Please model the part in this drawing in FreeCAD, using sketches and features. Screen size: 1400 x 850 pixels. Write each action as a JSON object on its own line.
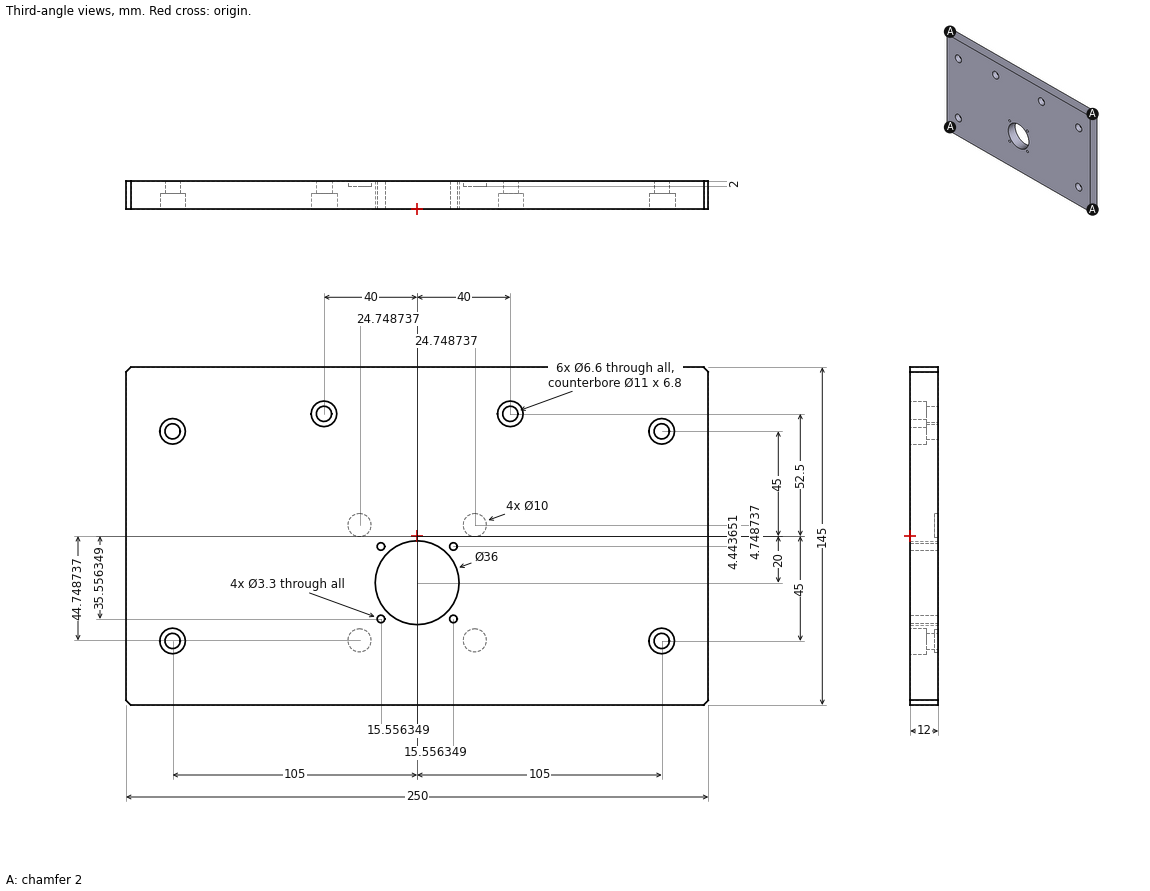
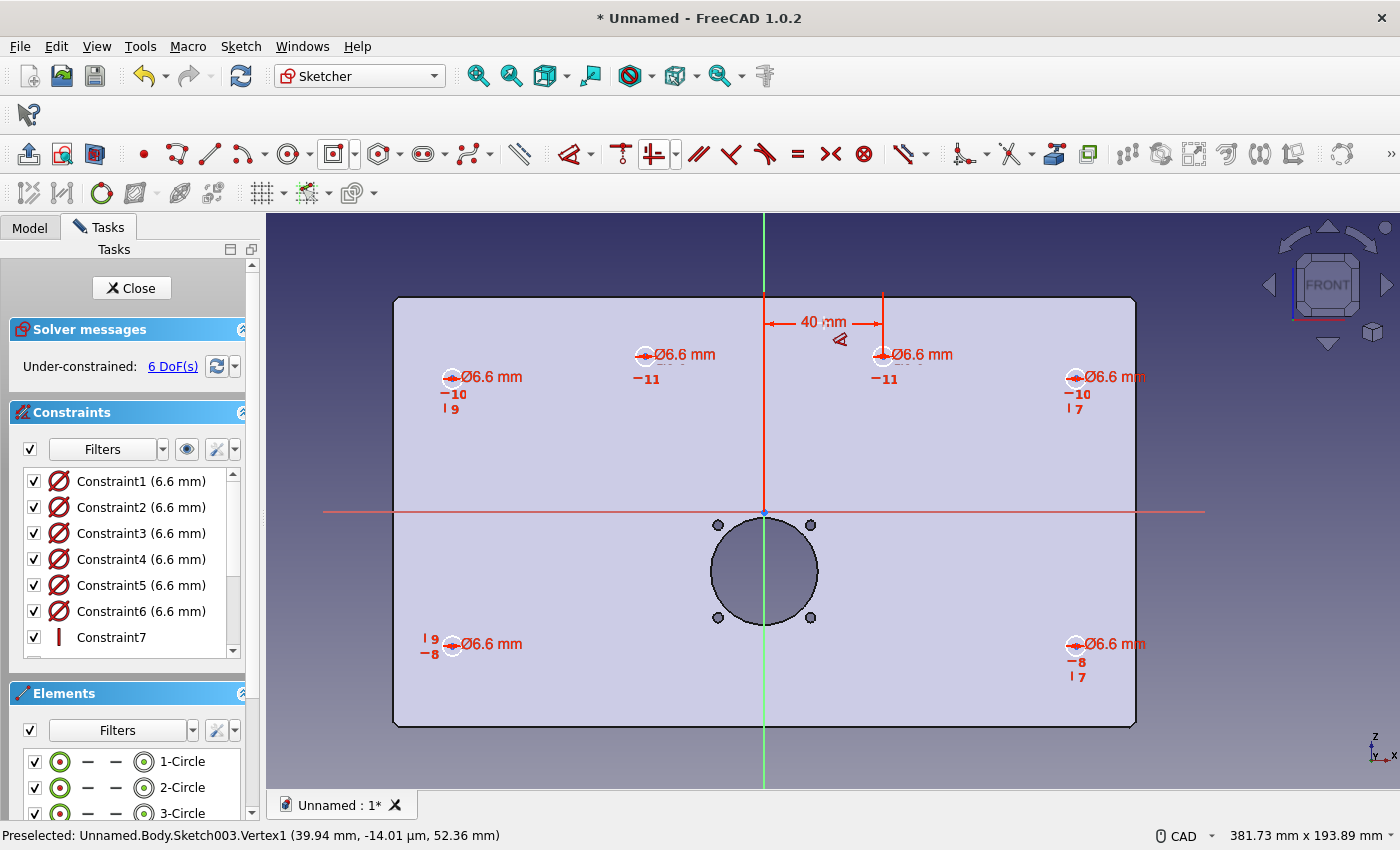
{"action": "left_click", "coordinate": [1076, 646]}
{"action": "left_click", "coordinate": [1110, 579]}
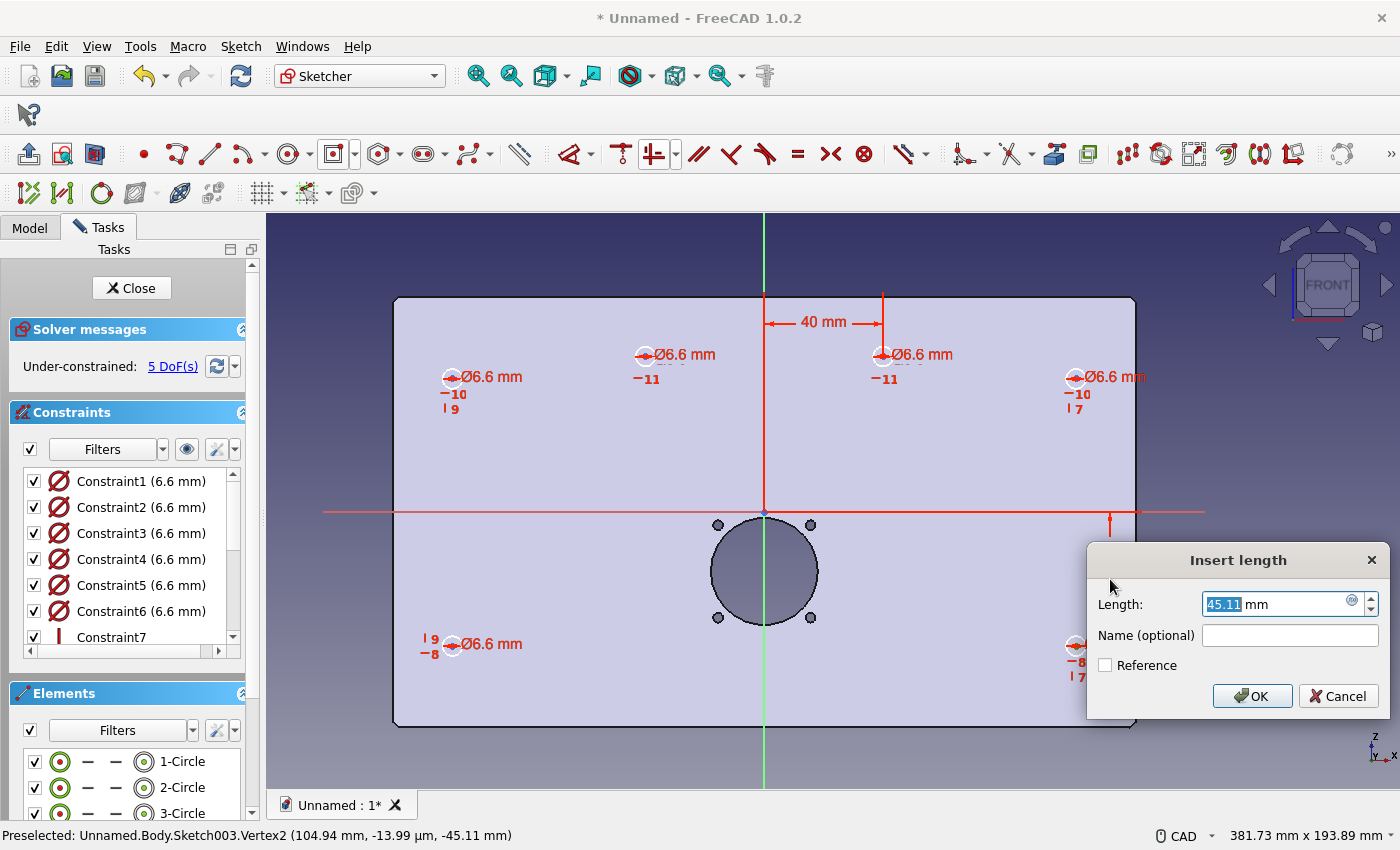
{"action": "type", "text": "45"}
{"action": "key", "text": "Return"}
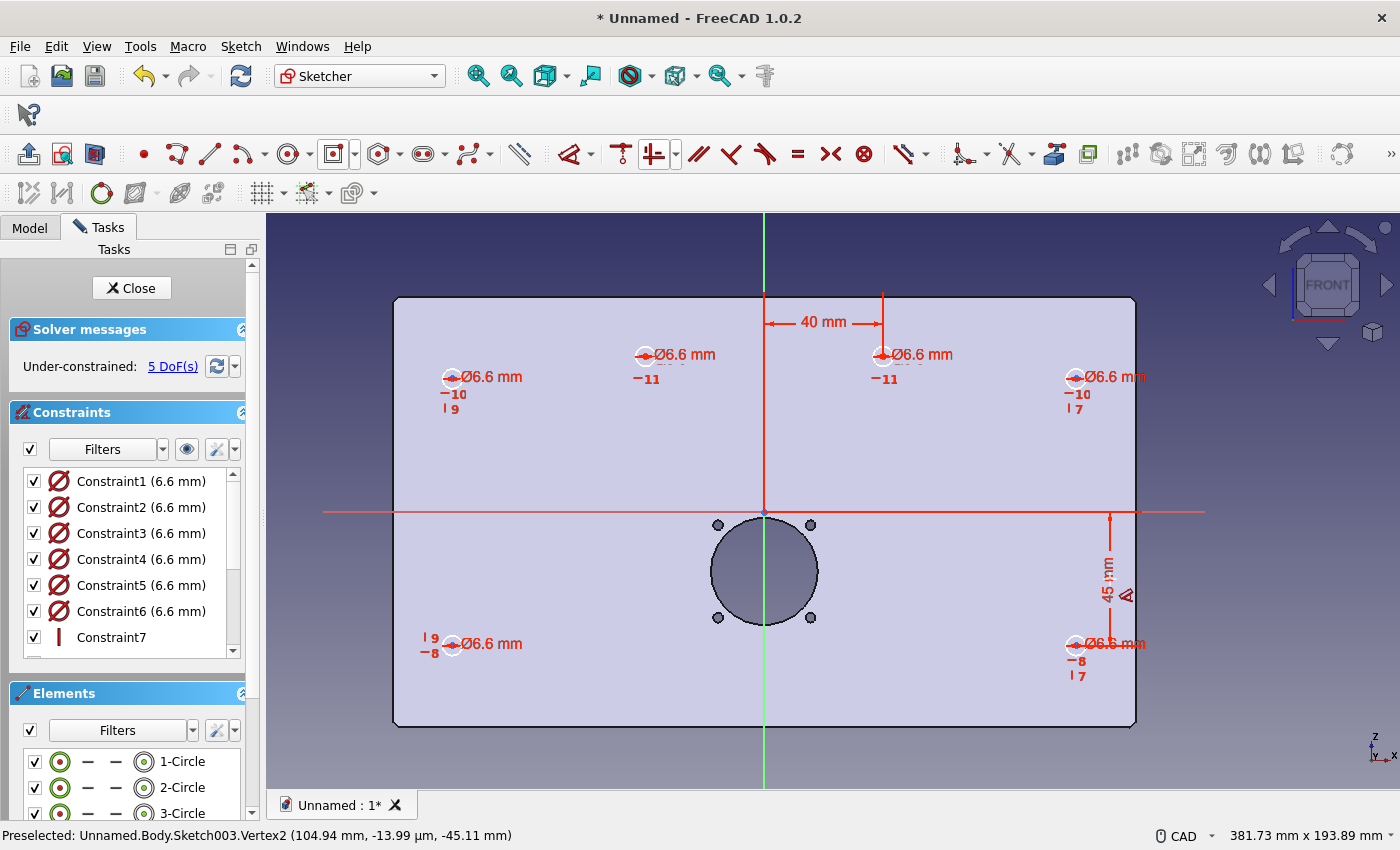
{"action": "left_click", "coordinate": [1076, 379]}
{"action": "left_click", "coordinate": [1110, 446]}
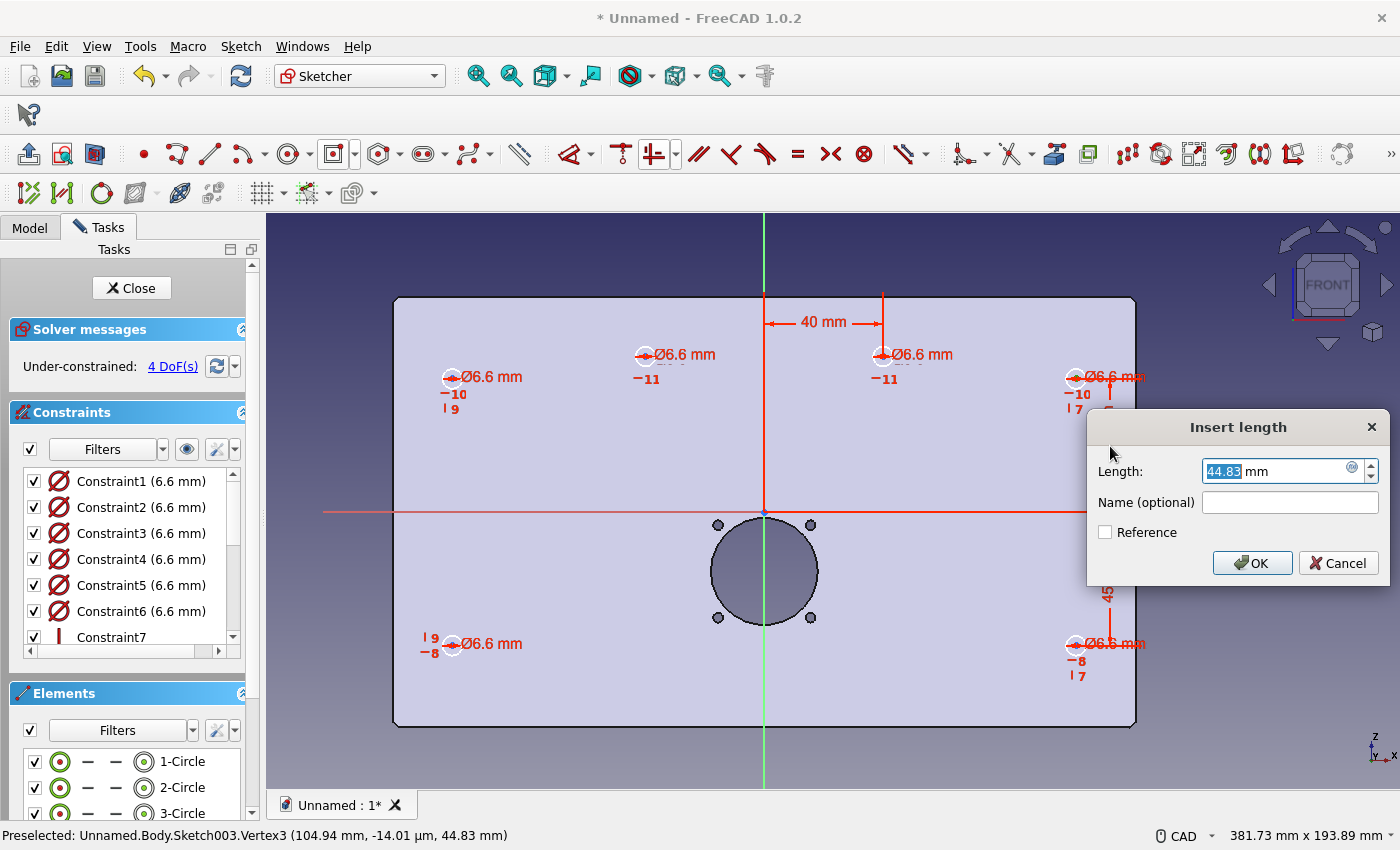
{"action": "type", "text": "45"}
{"action": "key", "text": "Return"}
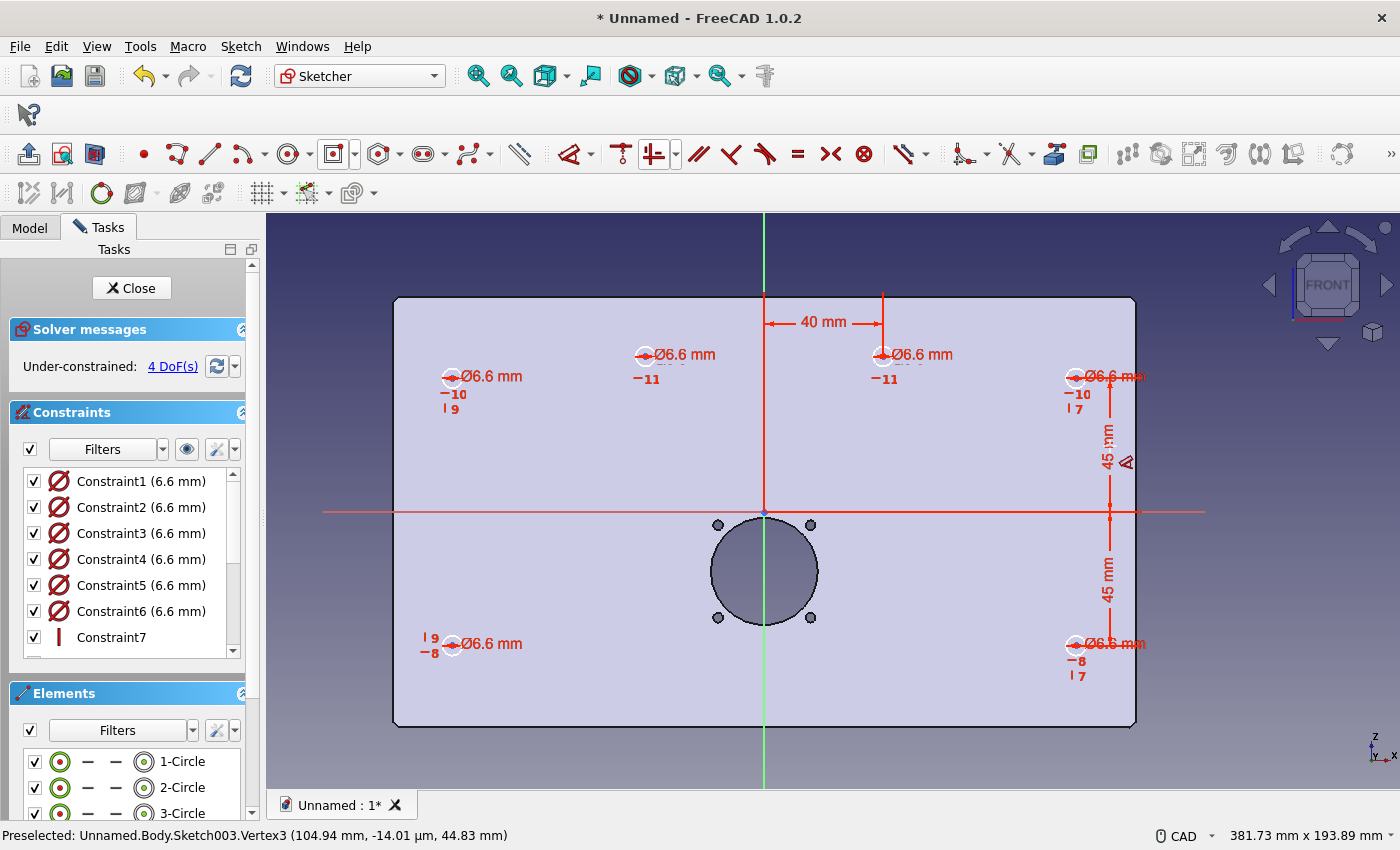
{"action": "left_click", "coordinate": [646, 357]}
{"action": "left_click", "coordinate": [705, 323]}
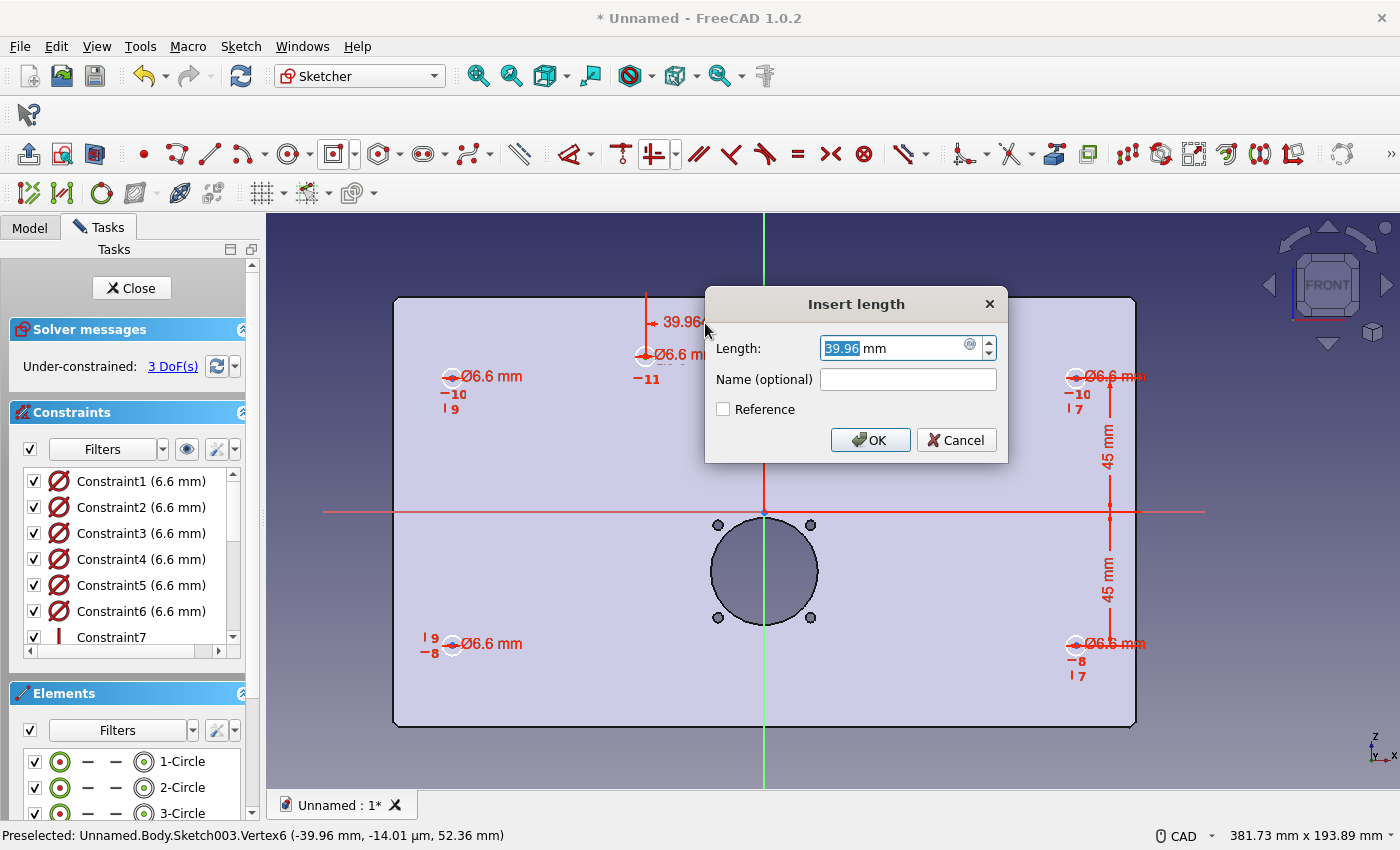
{"action": "type", "text": "40"}
{"action": "key", "text": "Return"}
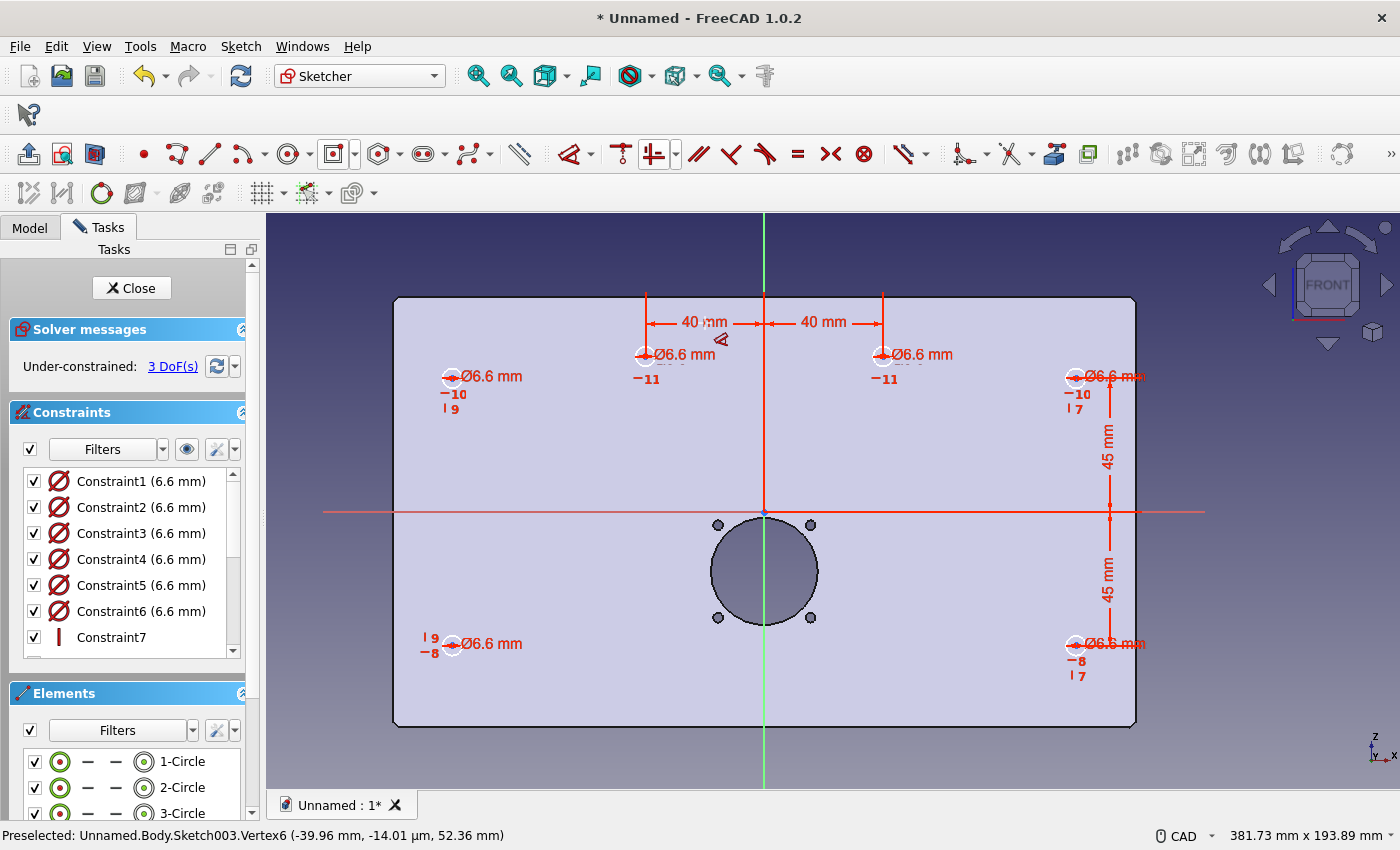
{"action": "left_click", "coordinate": [1076, 646]}
{"action": "left_click", "coordinate": [920, 680]}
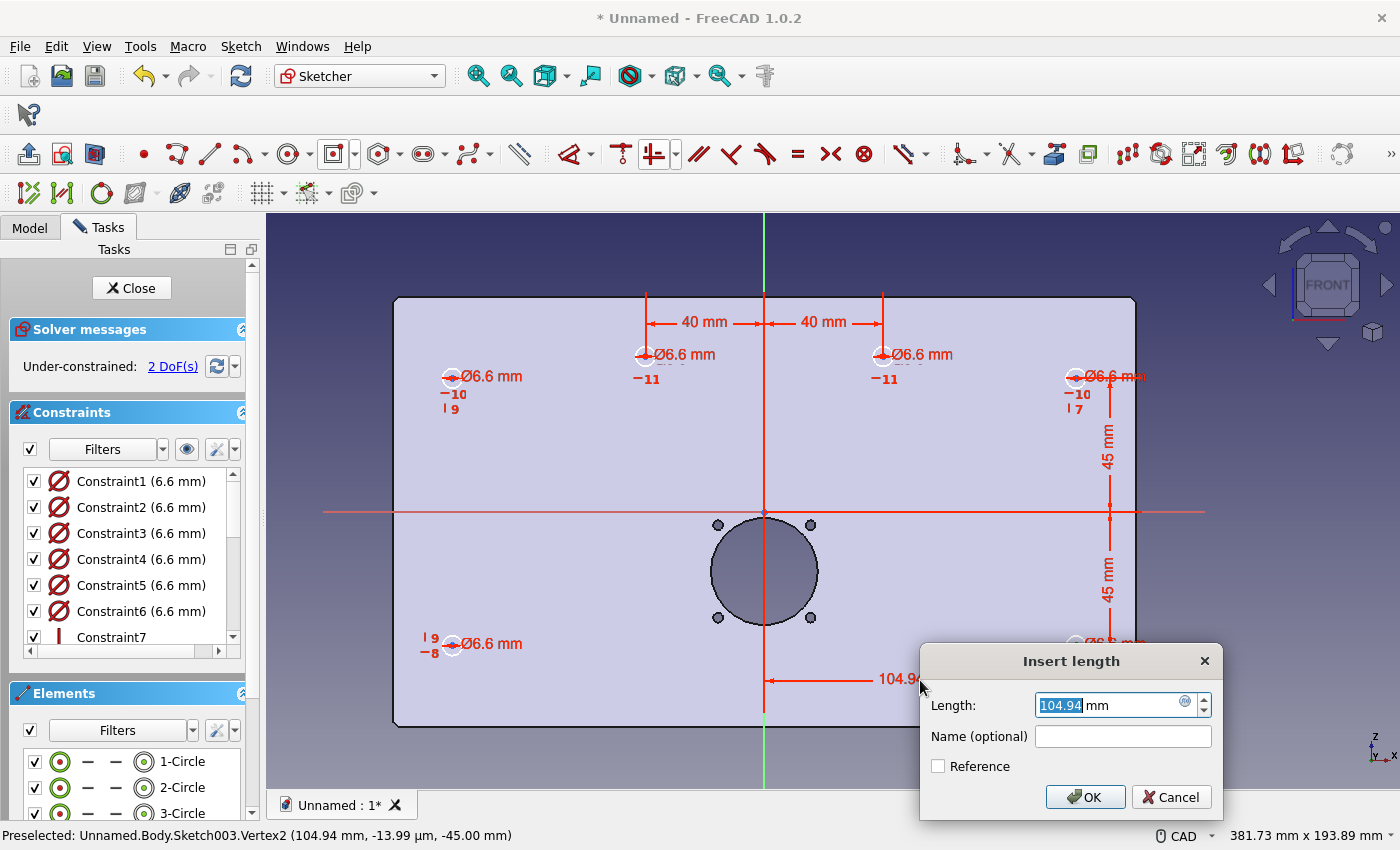
{"action": "type", "text": "105"}
{"action": "key", "text": "Return"}